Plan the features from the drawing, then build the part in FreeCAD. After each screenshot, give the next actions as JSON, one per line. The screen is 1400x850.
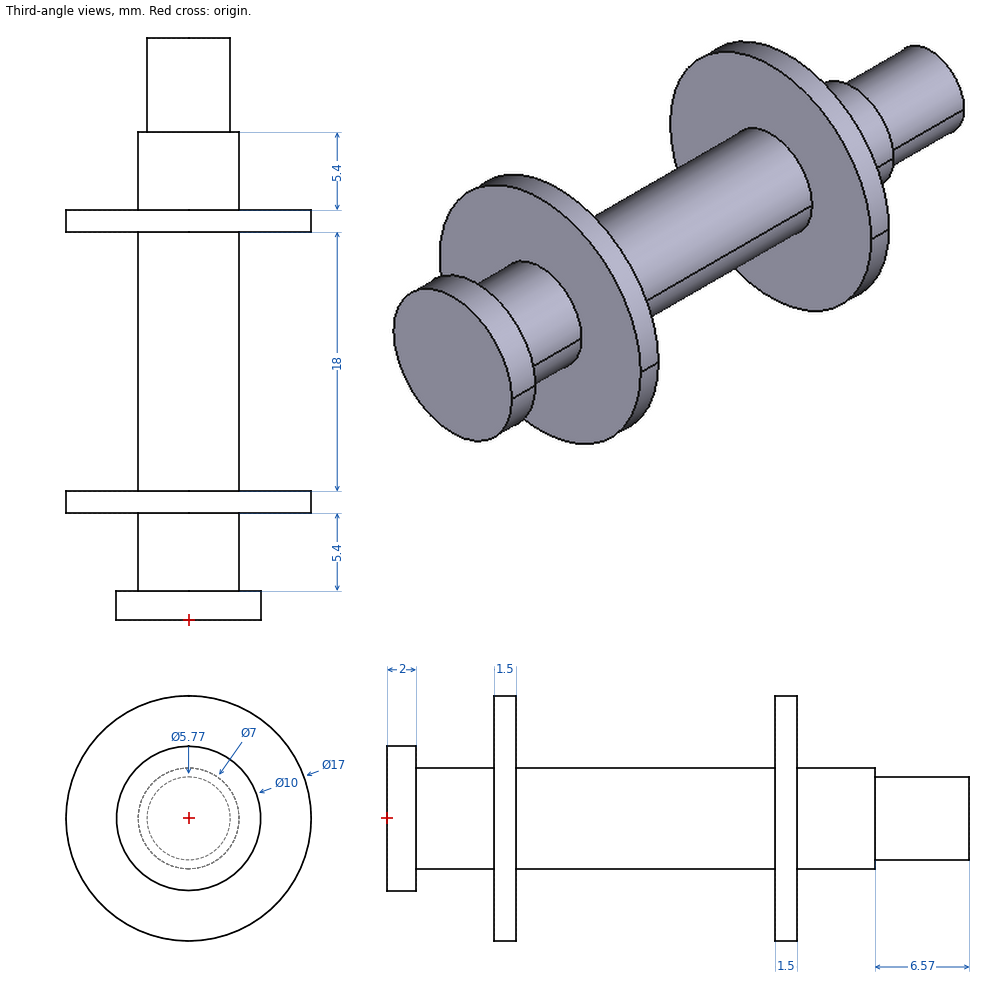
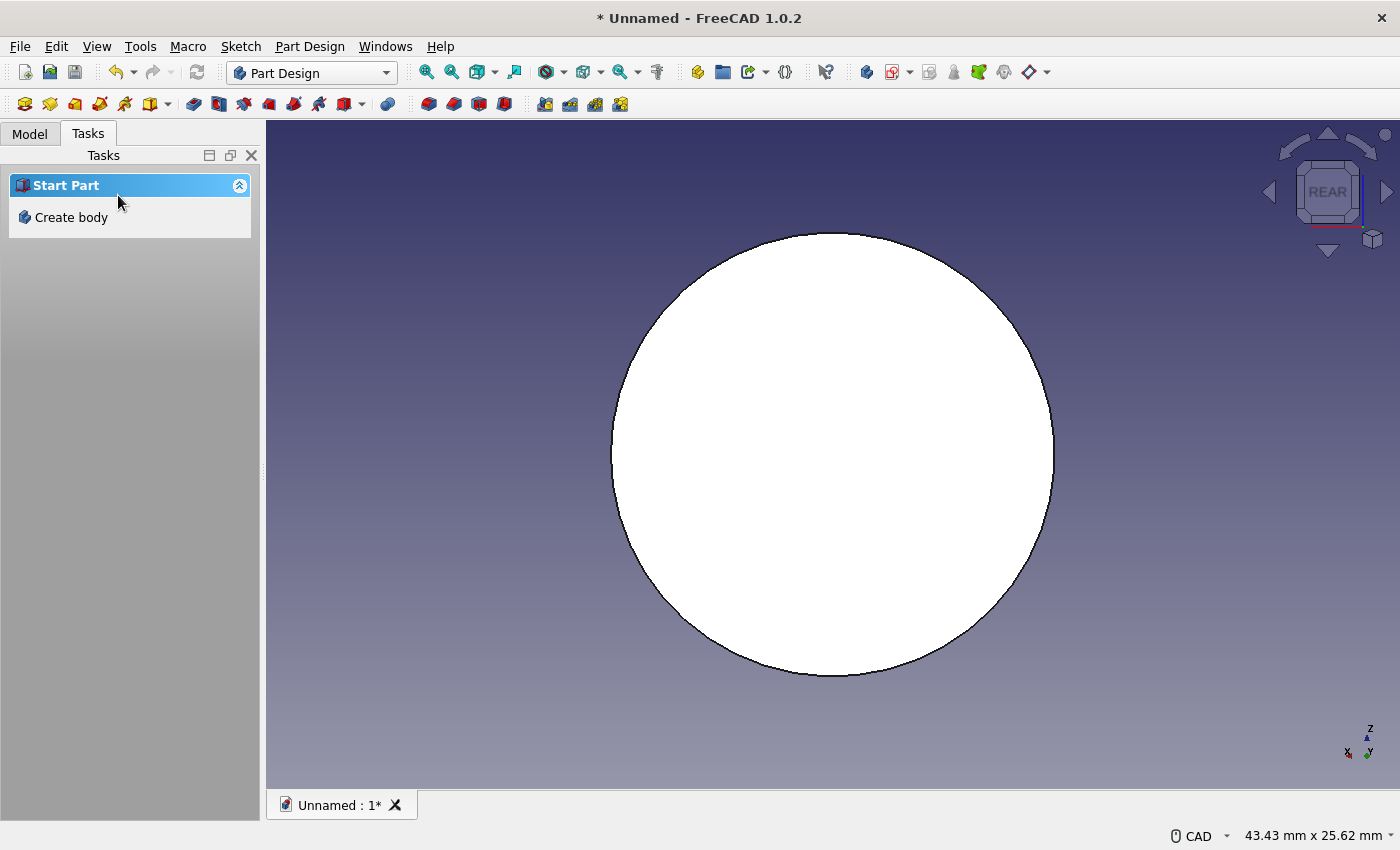
{"action": "left_click", "coordinate": [833, 453]}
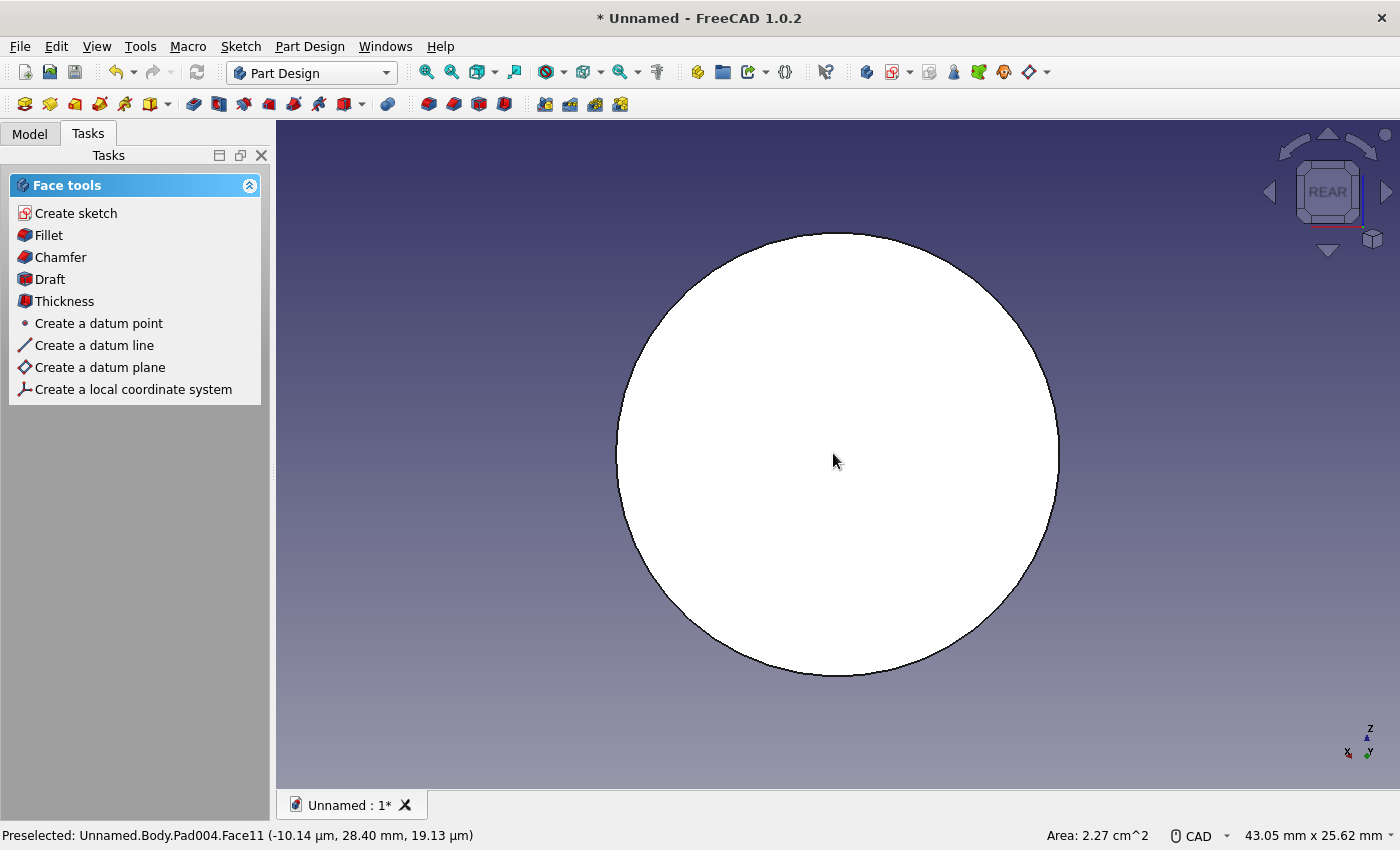
{"action": "left_click", "coordinate": [892, 72]}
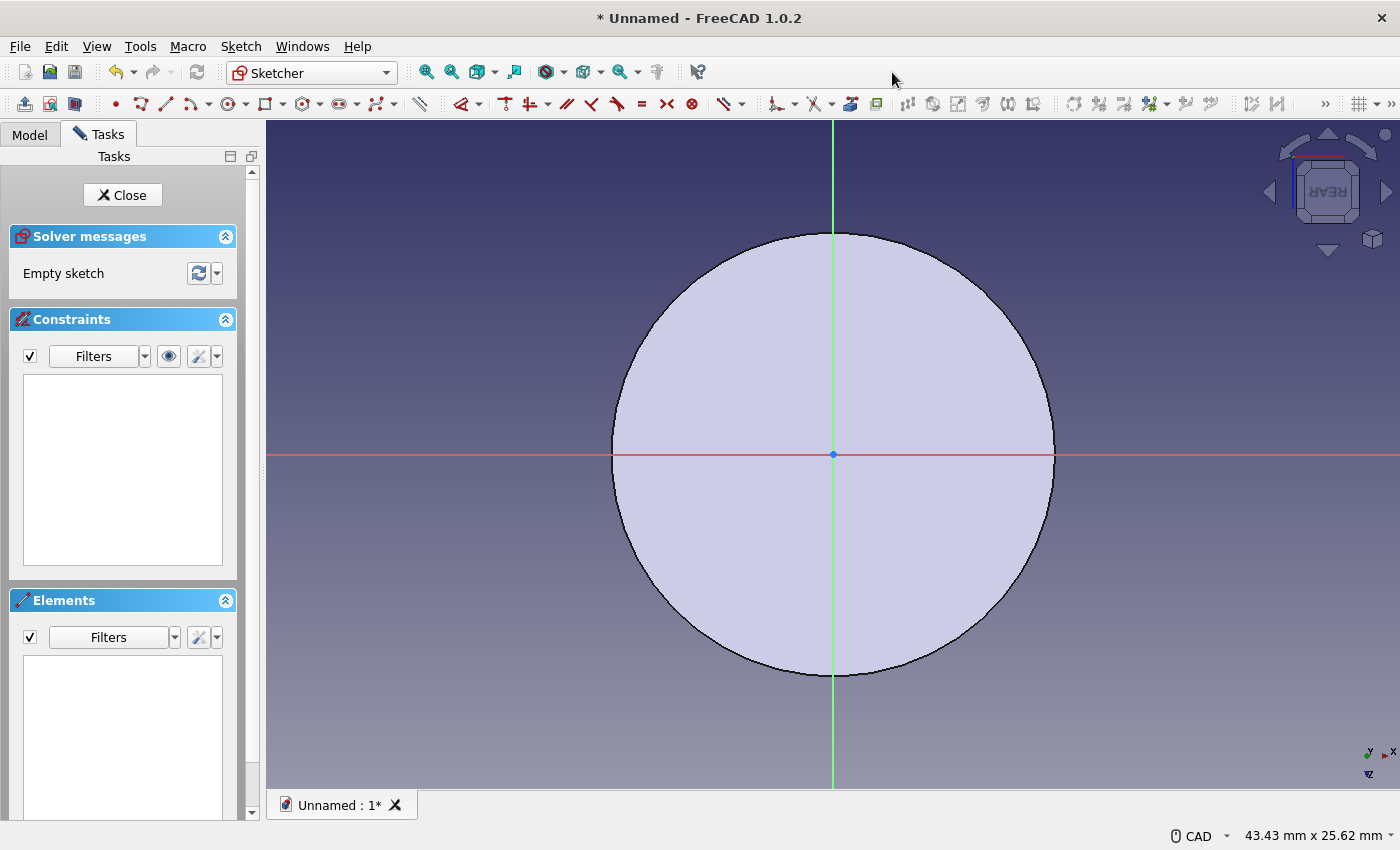
{"action": "scroll", "coordinate": [889, 455], "scroll_direction": "up", "scroll_amount": 4}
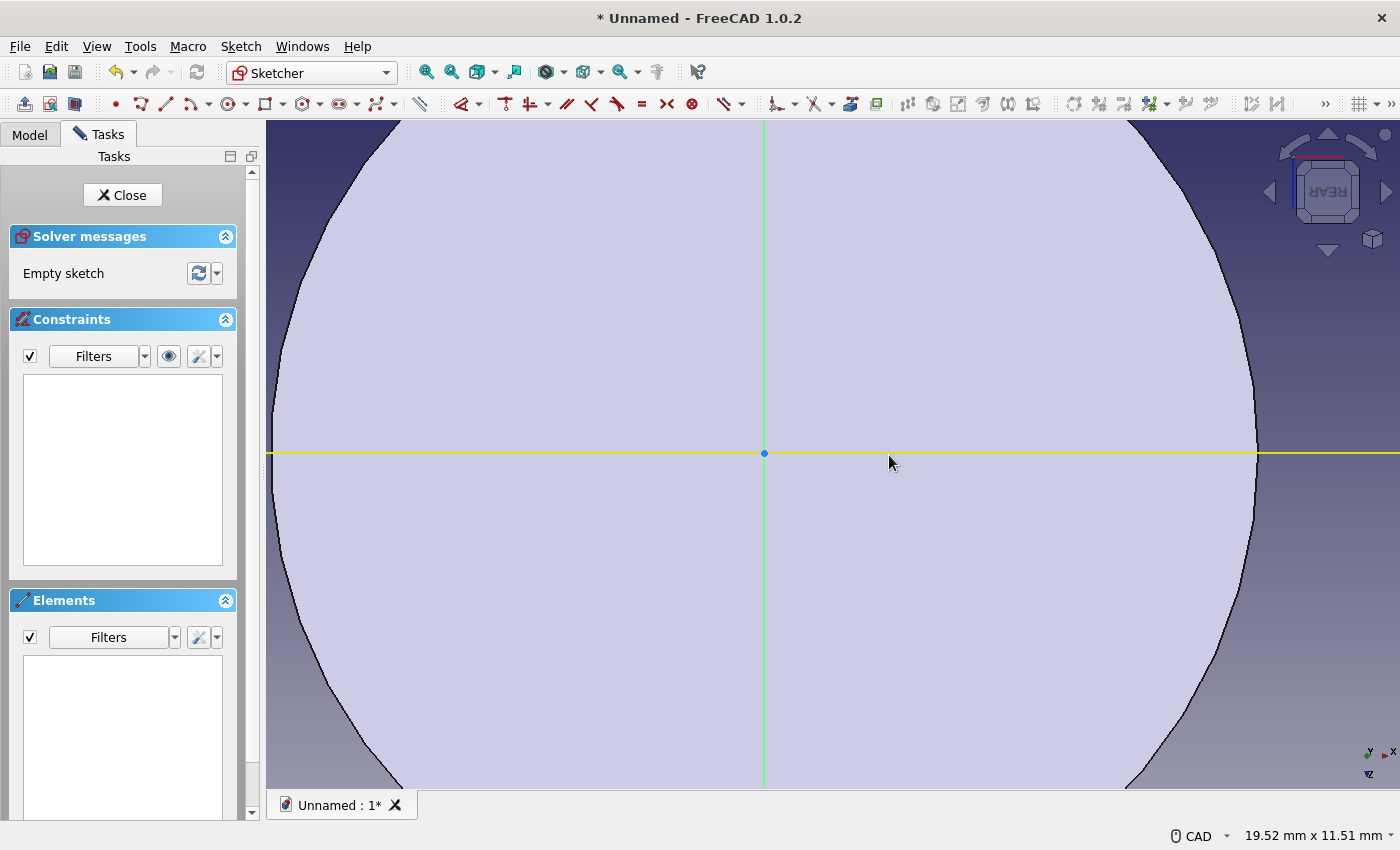
{"action": "left_click", "coordinate": [228, 104]}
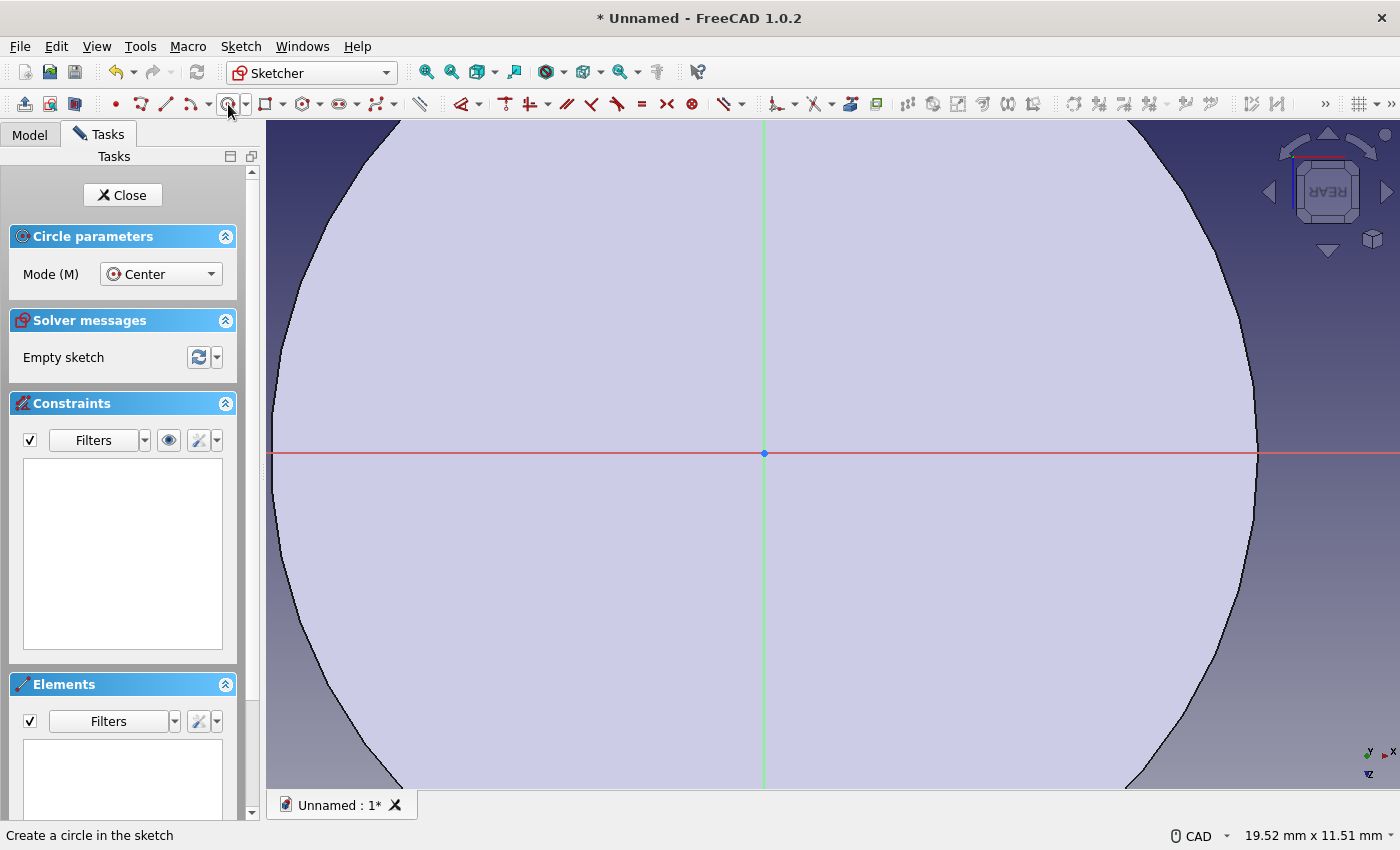
{"action": "left_click", "coordinate": [764, 453]}
{"action": "left_click", "coordinate": [908, 309]}
{"action": "key", "text": "Escape"}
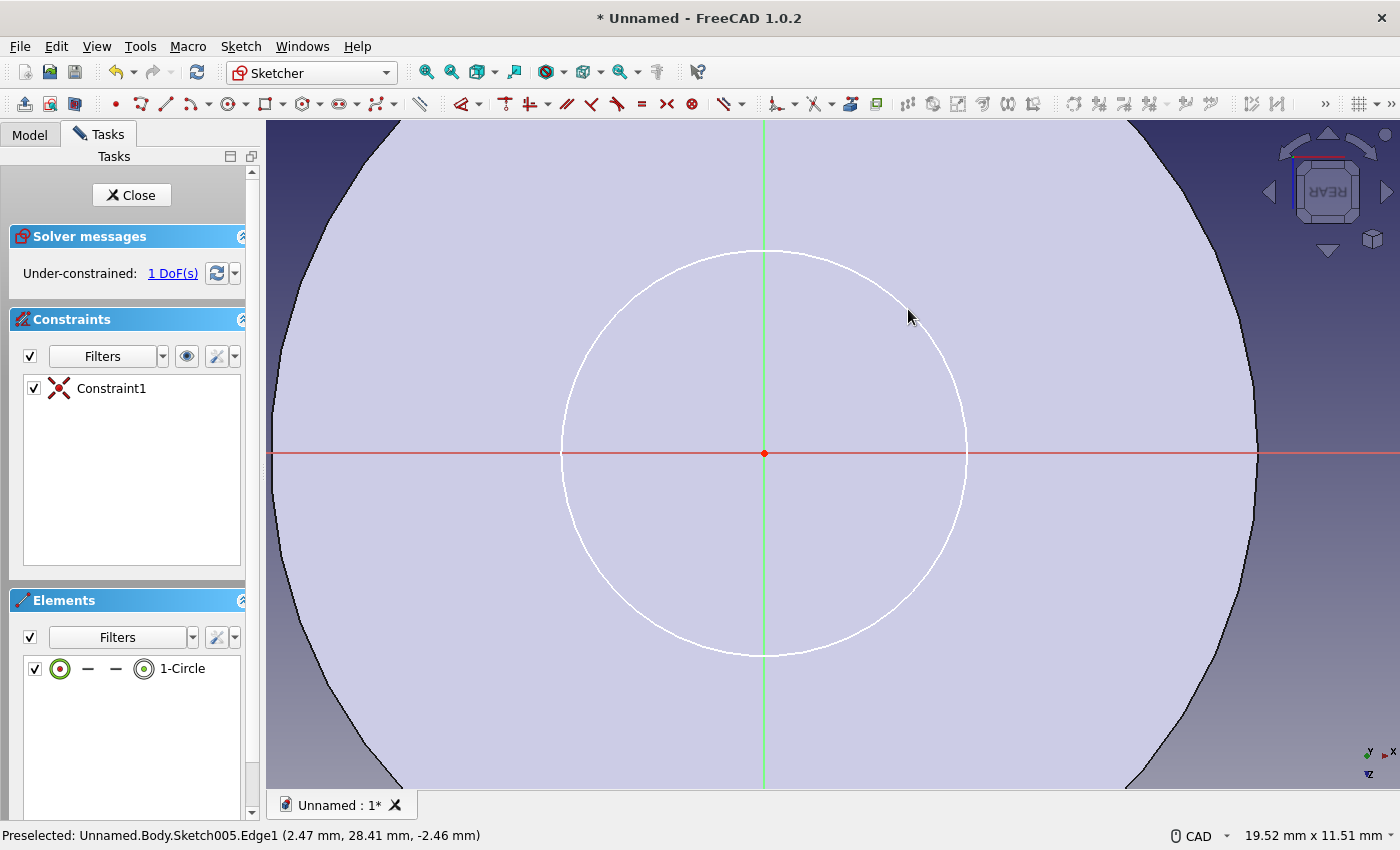
{"action": "left_click", "coordinate": [460, 104]}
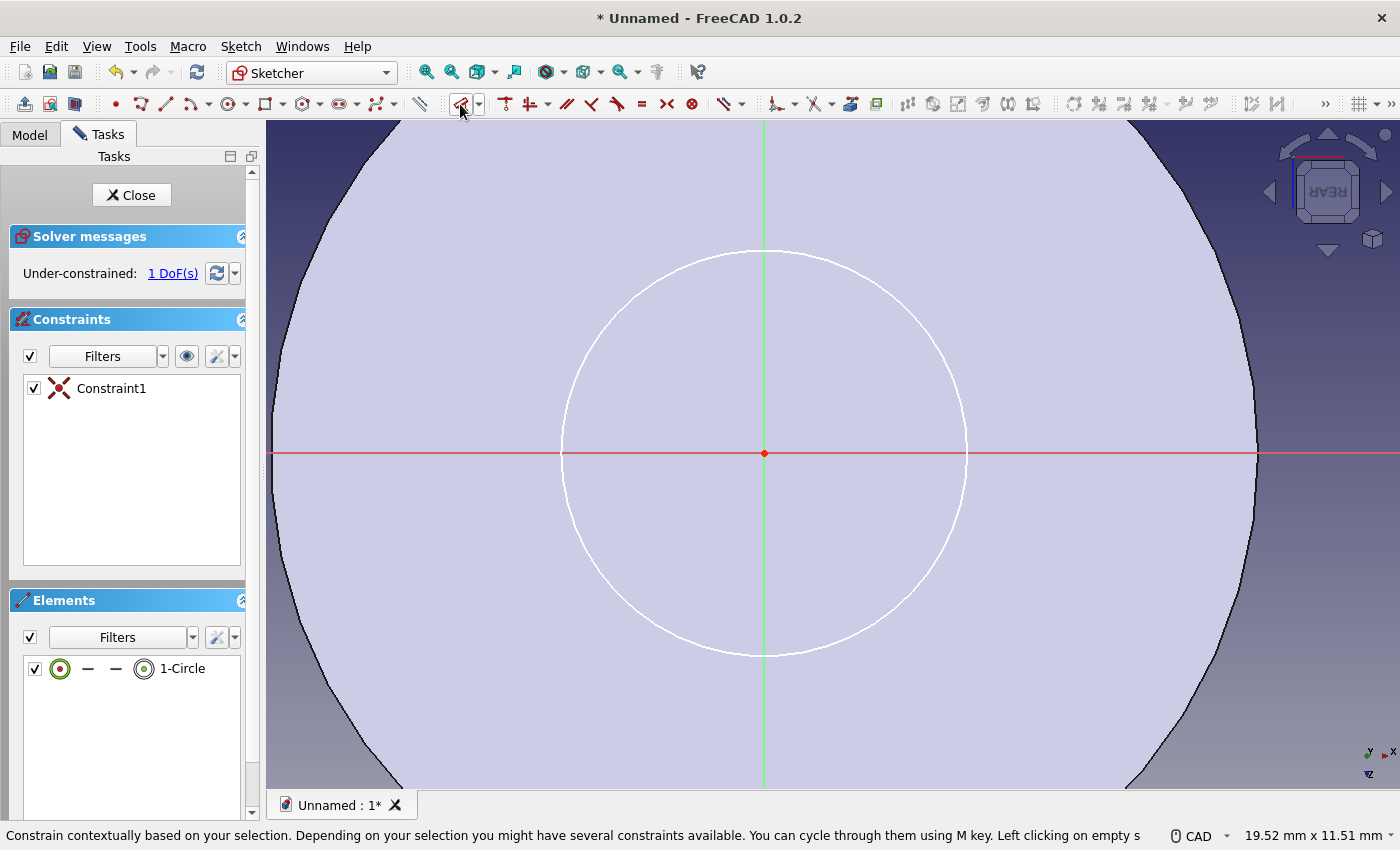
{"action": "left_click", "coordinate": [907, 309]}
{"action": "left_click", "coordinate": [930, 286]}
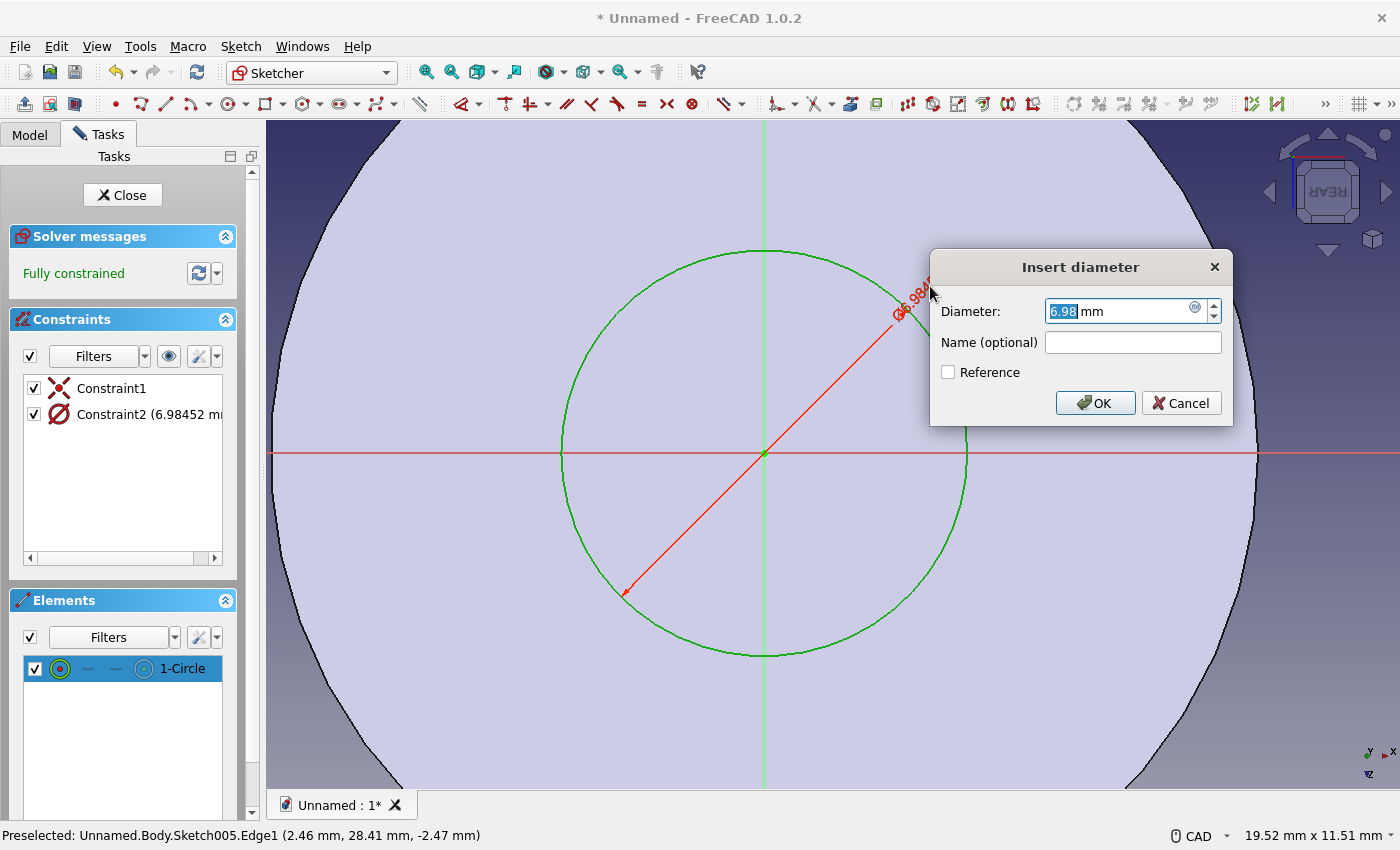
{"action": "type", "text": "7"}
{"action": "key", "text": "Return"}
{"action": "key", "text": "Escape"}